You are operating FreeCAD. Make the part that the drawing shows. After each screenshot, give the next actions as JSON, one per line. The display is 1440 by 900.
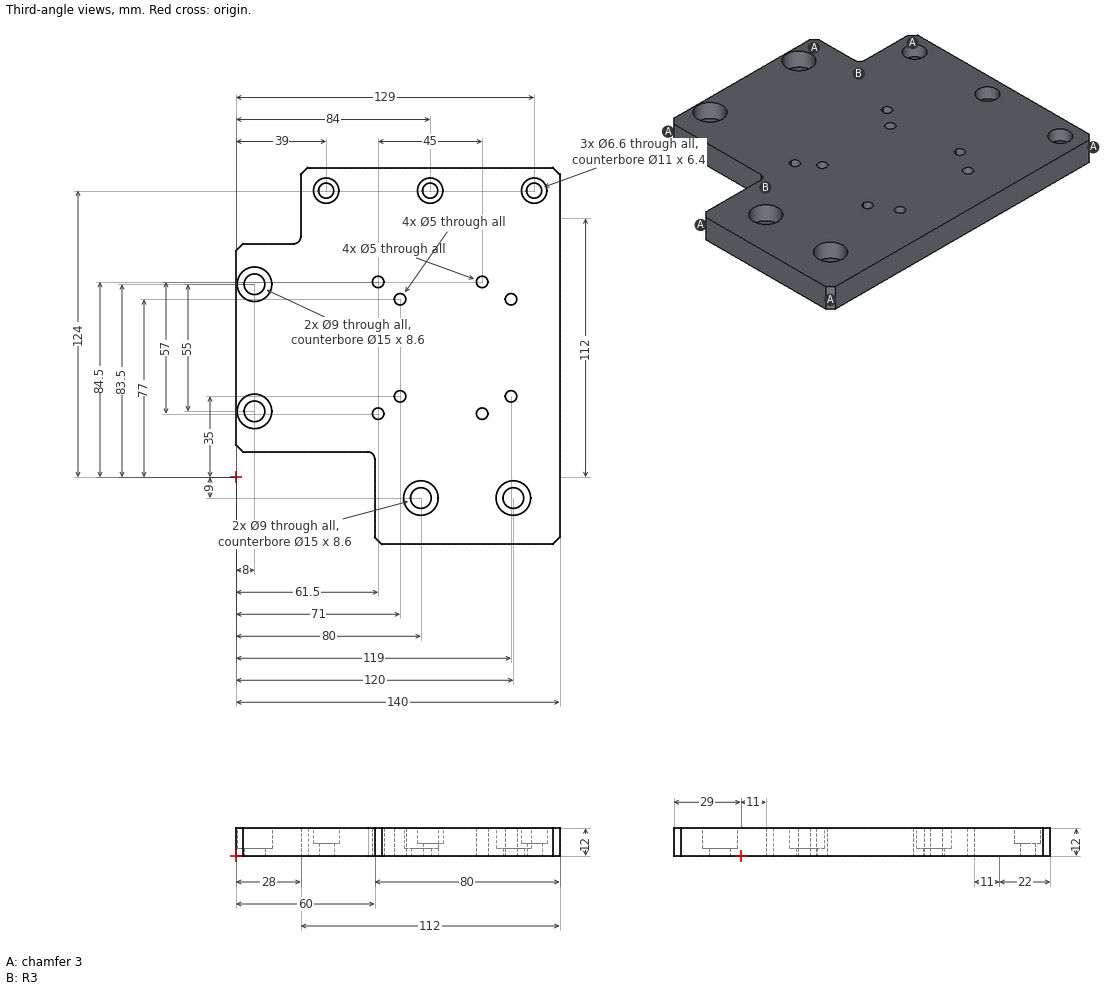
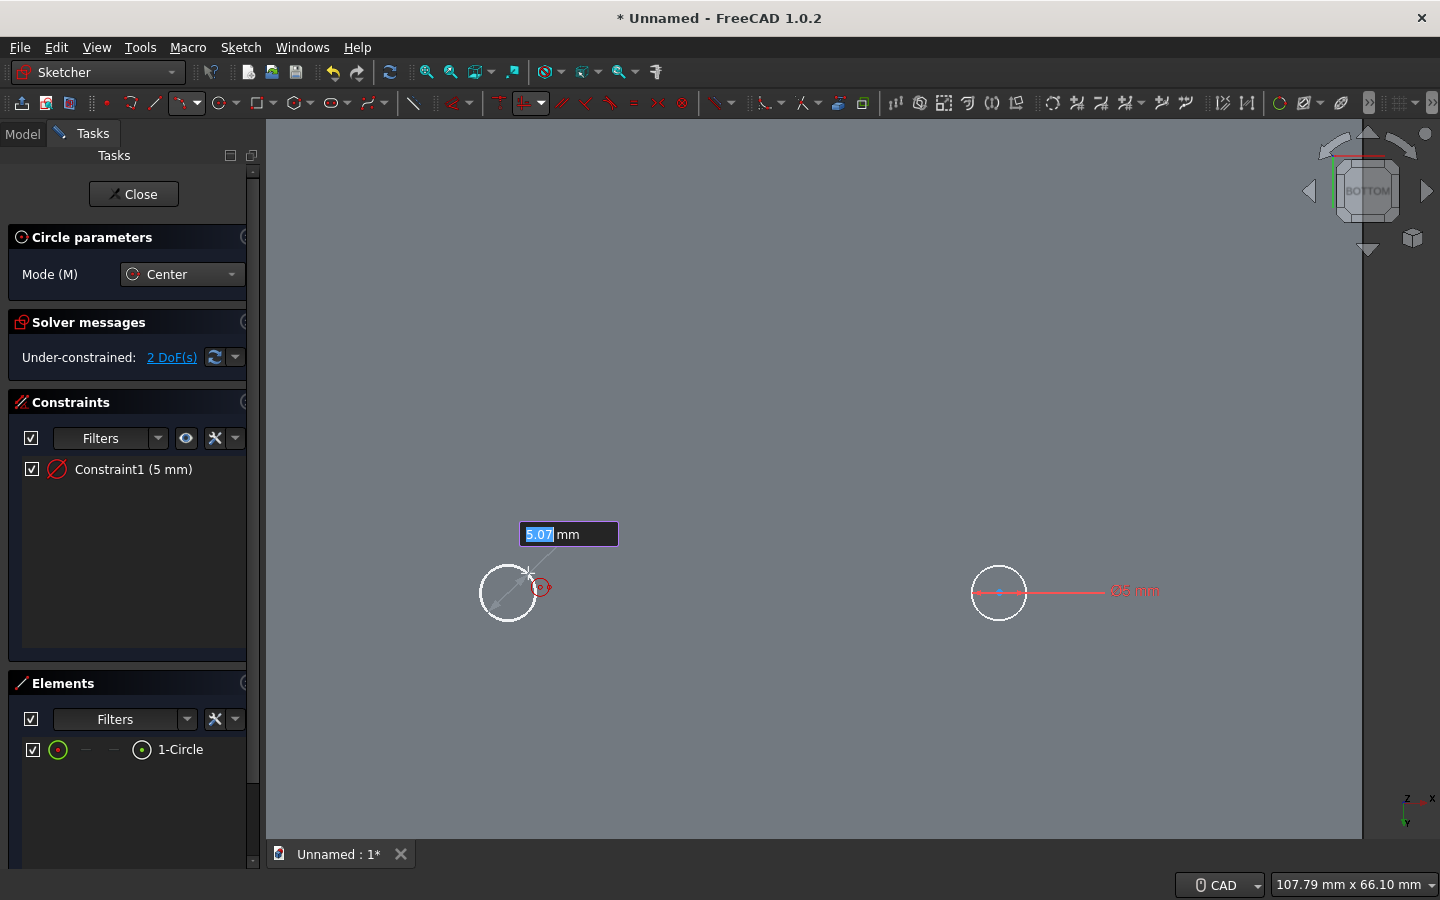
{"action": "type", "text": "5"}
{"action": "key", "text": "Return"}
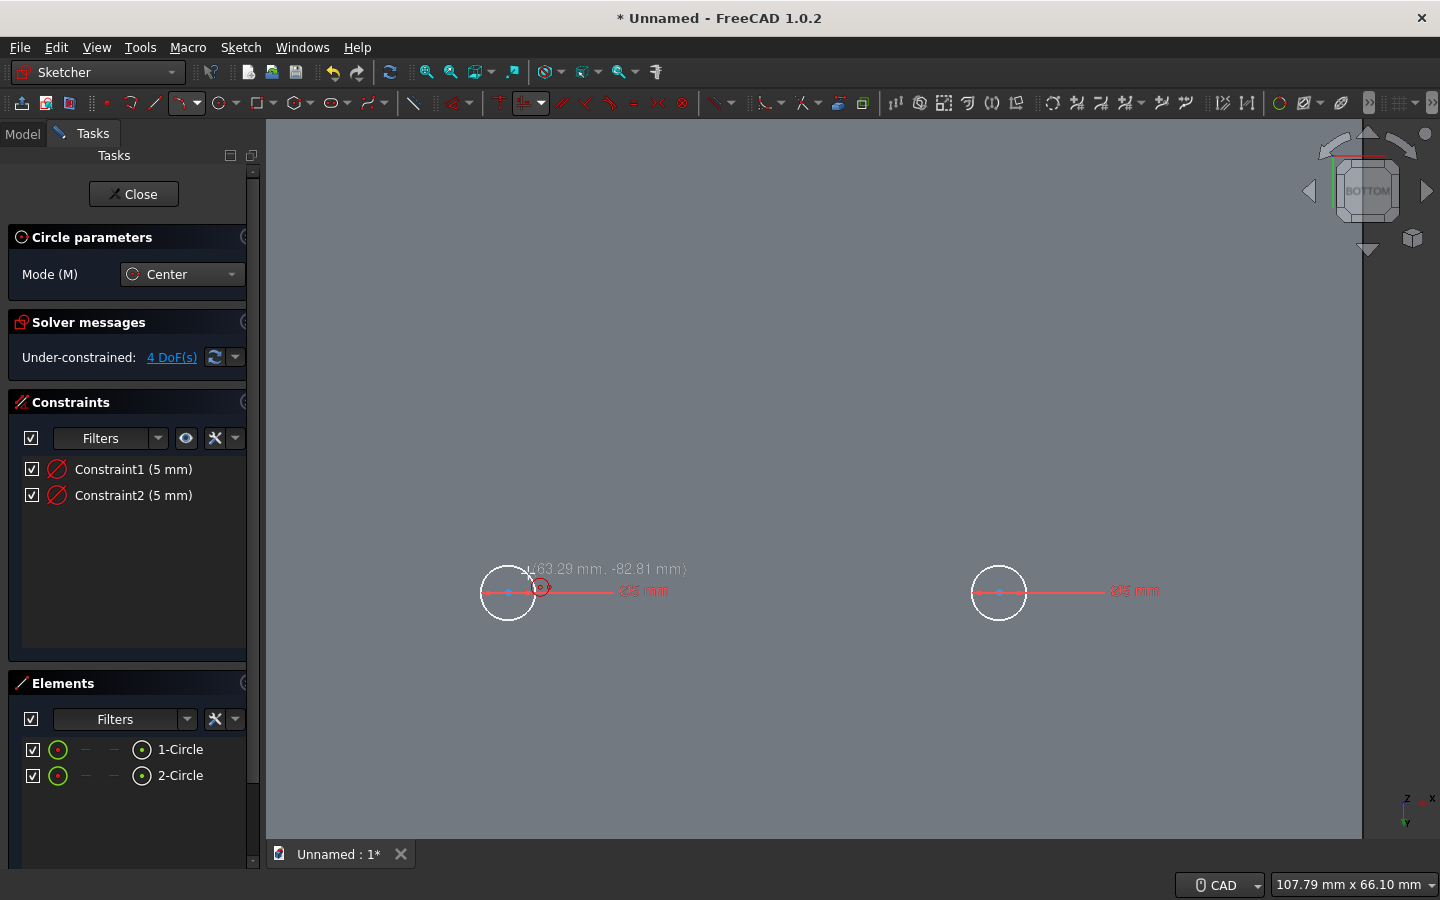
{"action": "scroll", "coordinate": [1072, 751], "scroll_direction": "down", "scroll_amount": 4}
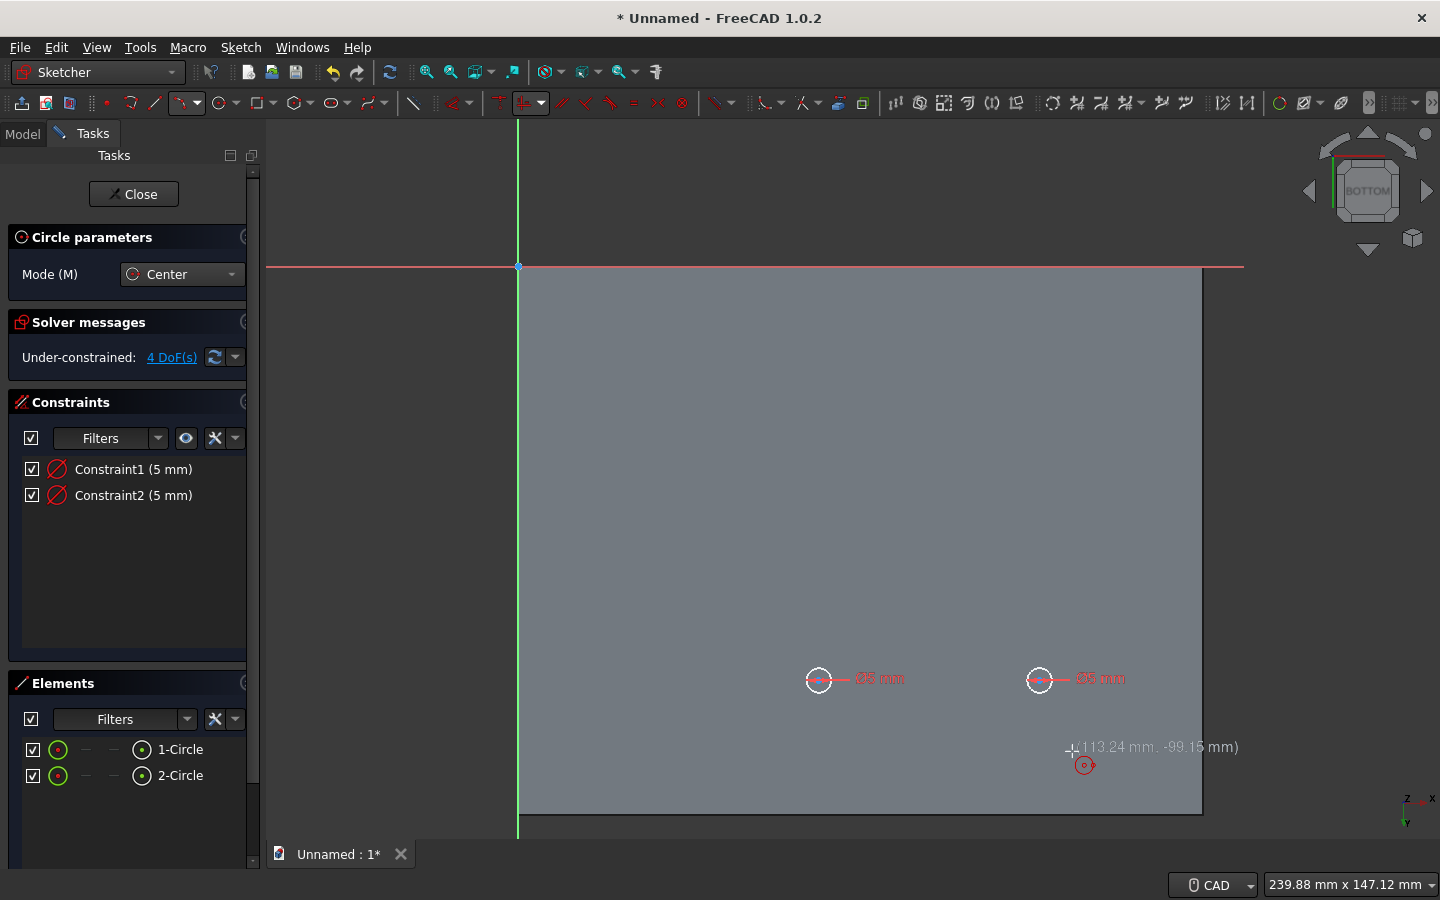
{"action": "scroll", "coordinate": [819, 401], "scroll_direction": "up", "scroll_amount": 4}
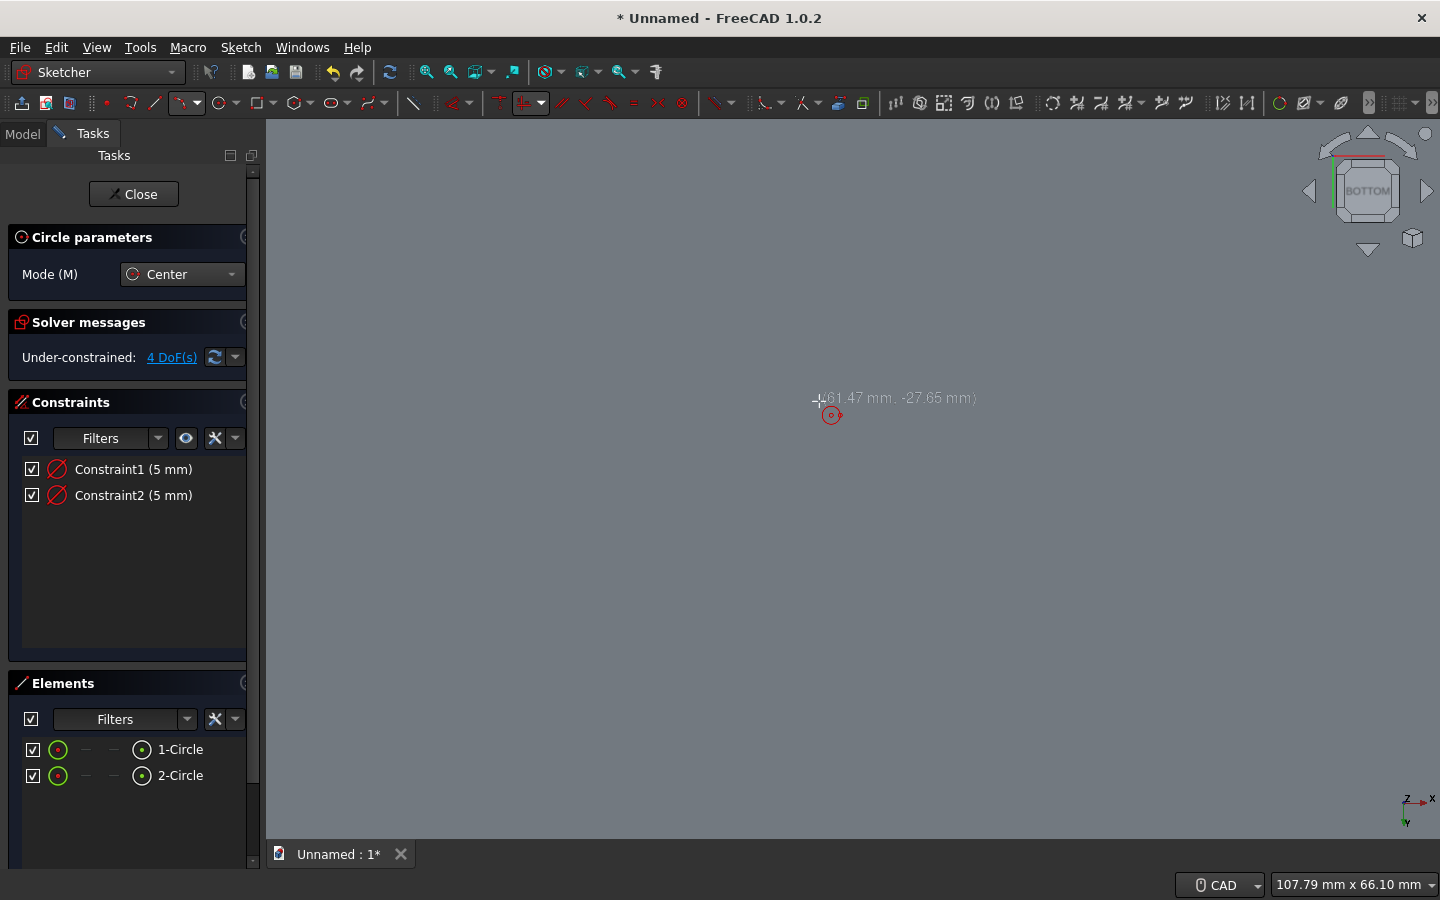
{"action": "left_click", "coordinate": [819, 401]}
{"action": "mouse_move", "coordinate": [838, 382]}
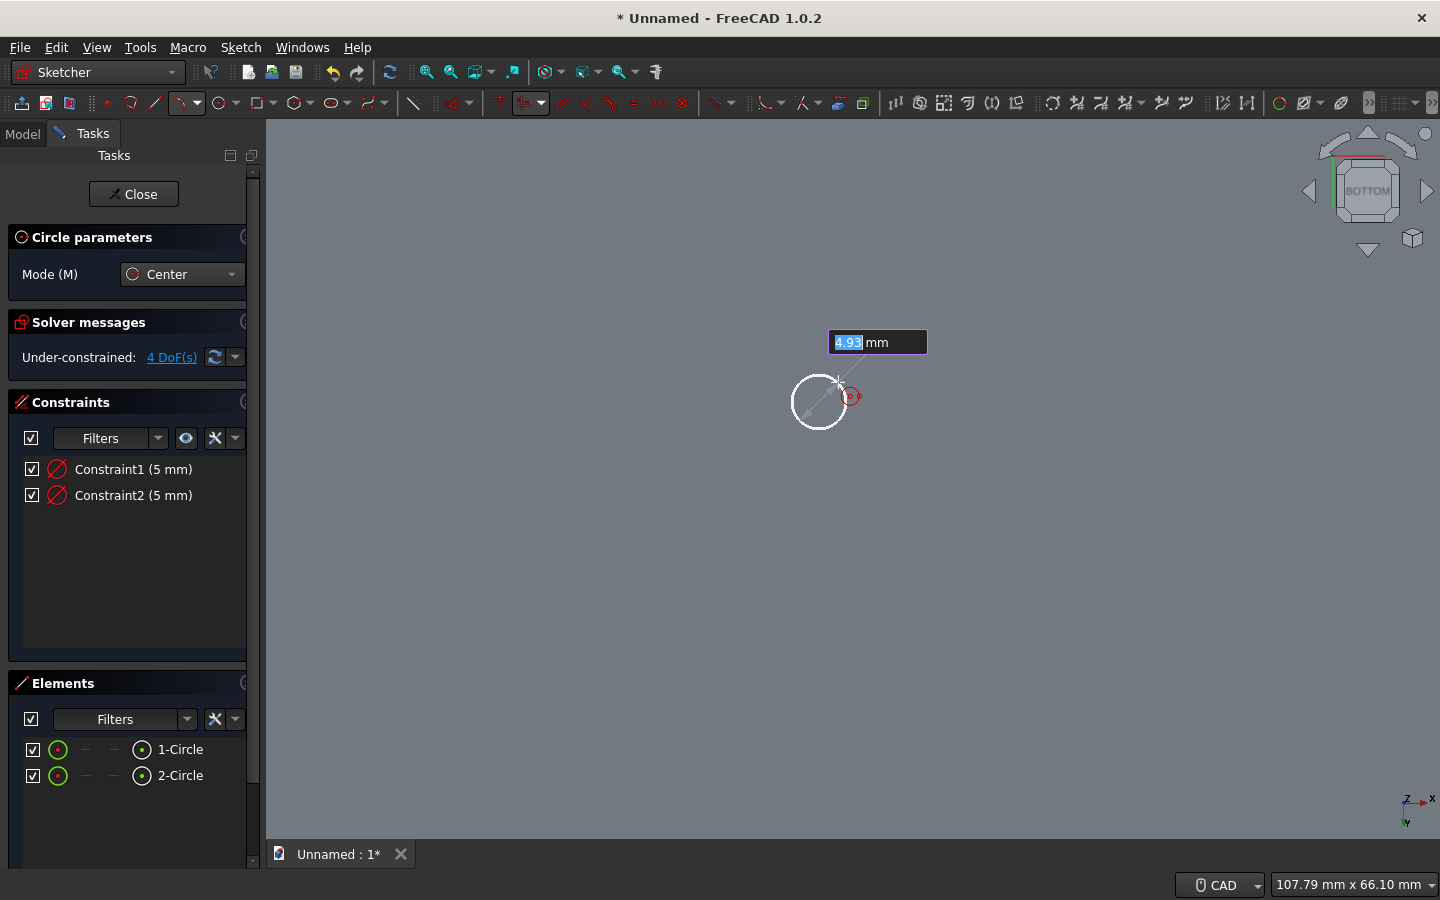
{"action": "type", "text": "5"}
{"action": "key", "text": "Return"}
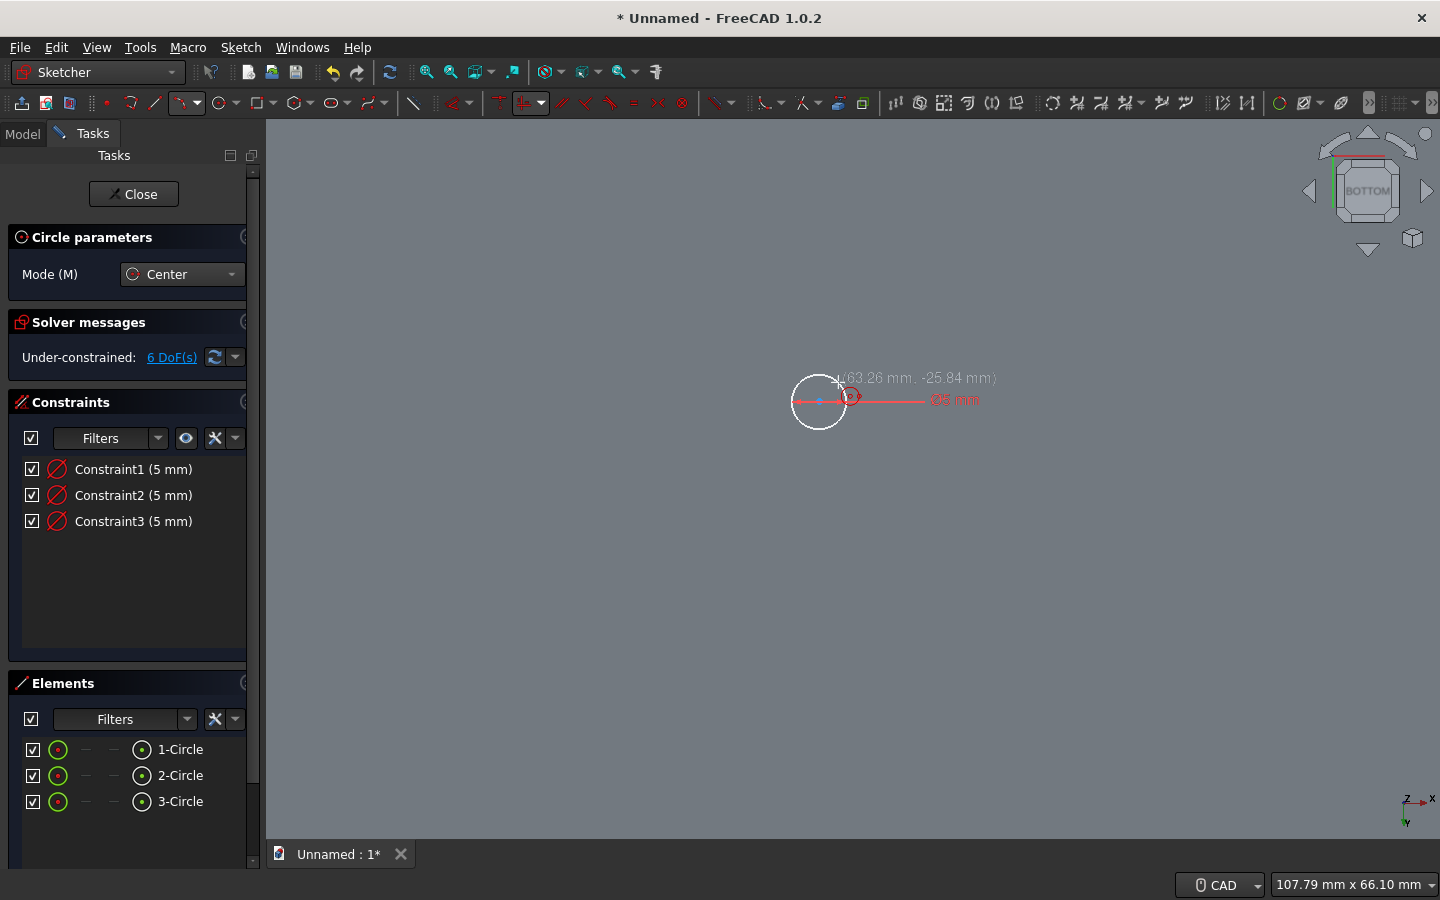
{"action": "scroll", "coordinate": [819, 400], "scroll_direction": "down", "scroll_amount": 4}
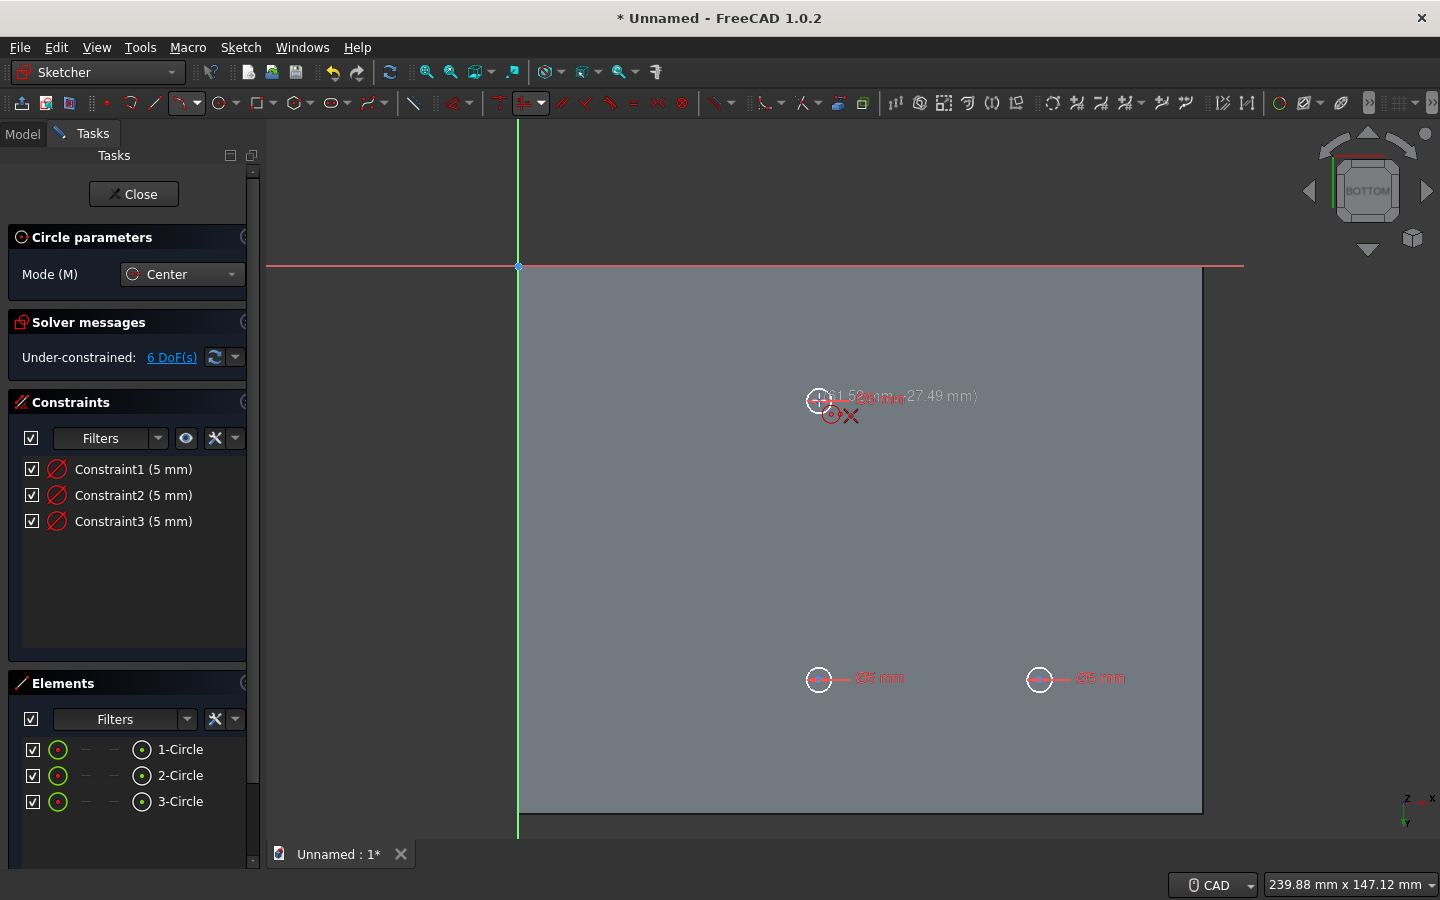
{"action": "scroll", "coordinate": [1039, 401], "scroll_direction": "up", "scroll_amount": 4}